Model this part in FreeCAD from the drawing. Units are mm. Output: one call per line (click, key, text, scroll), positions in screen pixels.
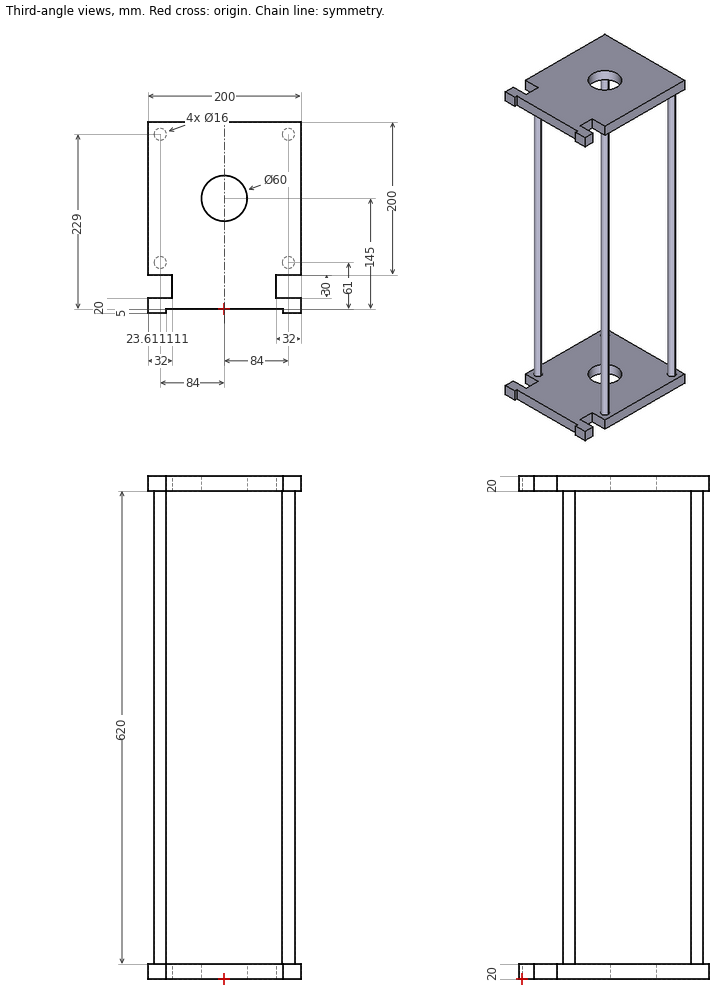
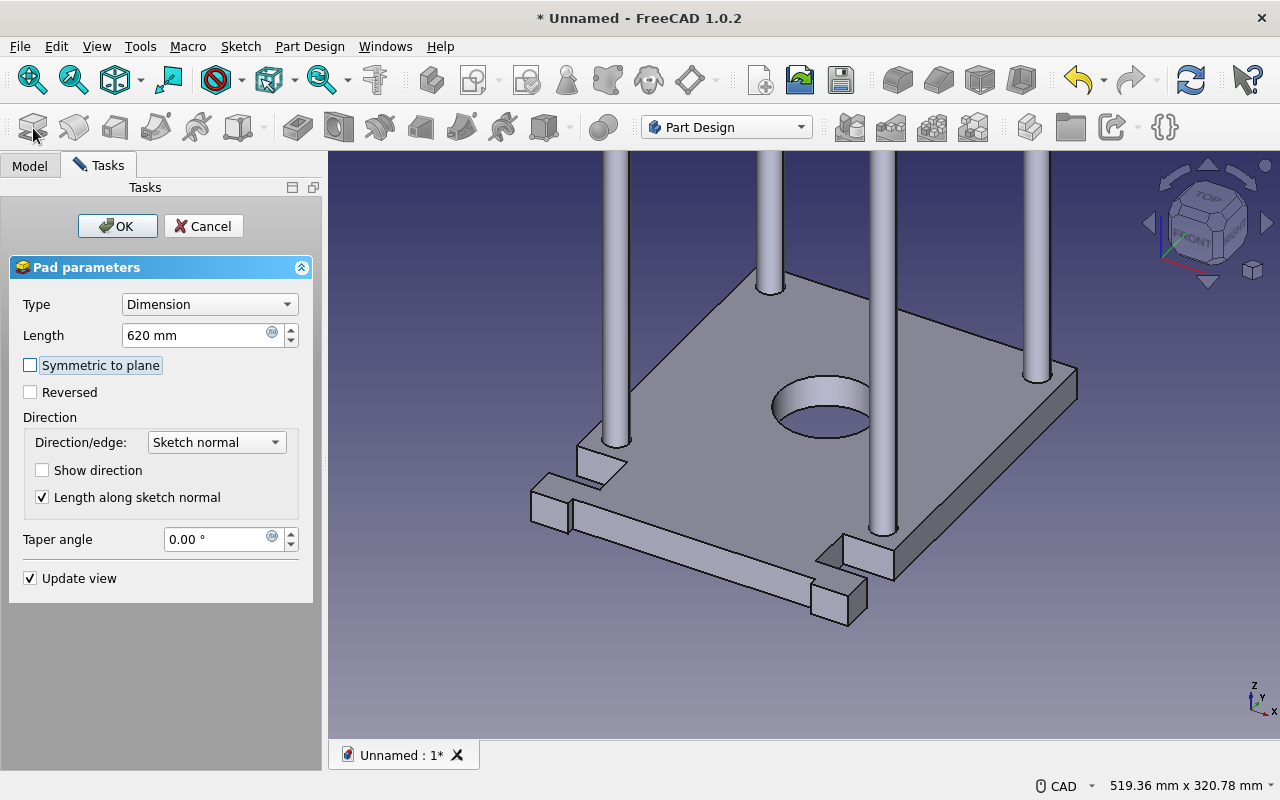
click(118, 226)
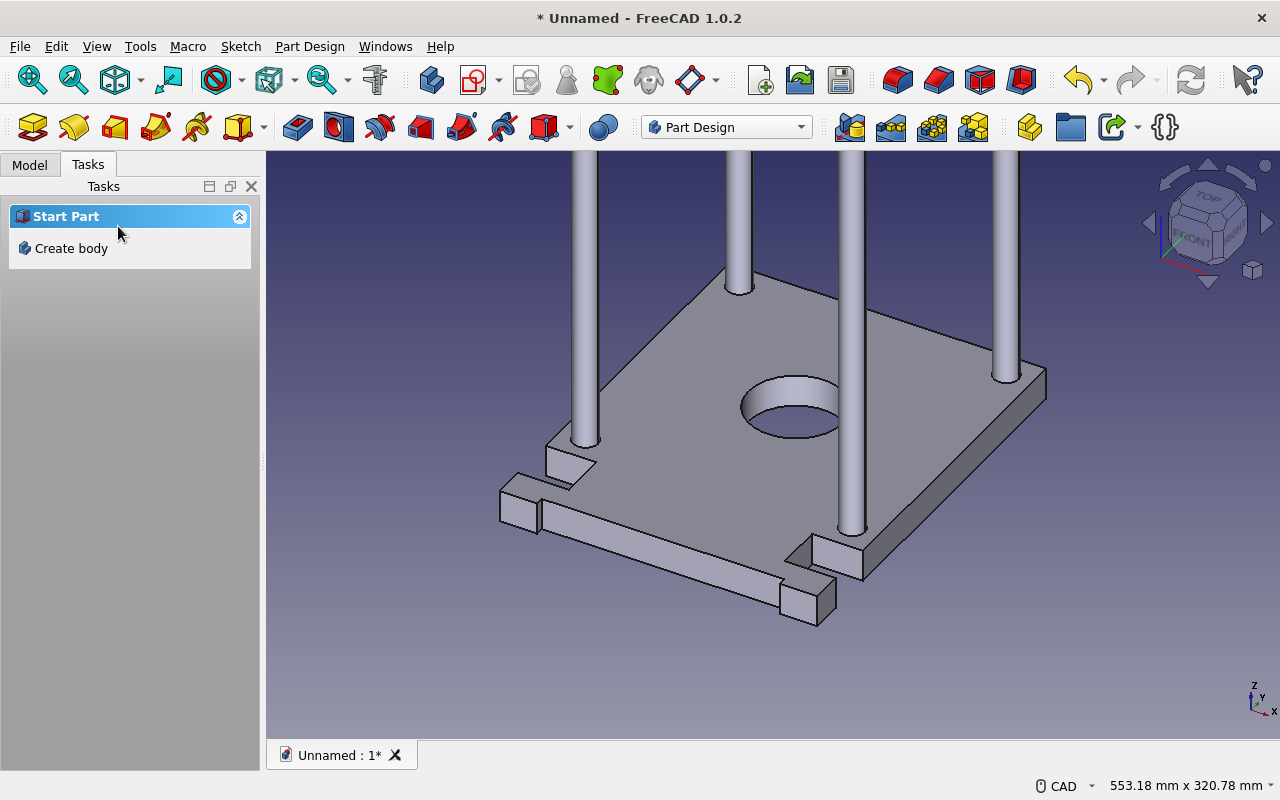
click(33, 80)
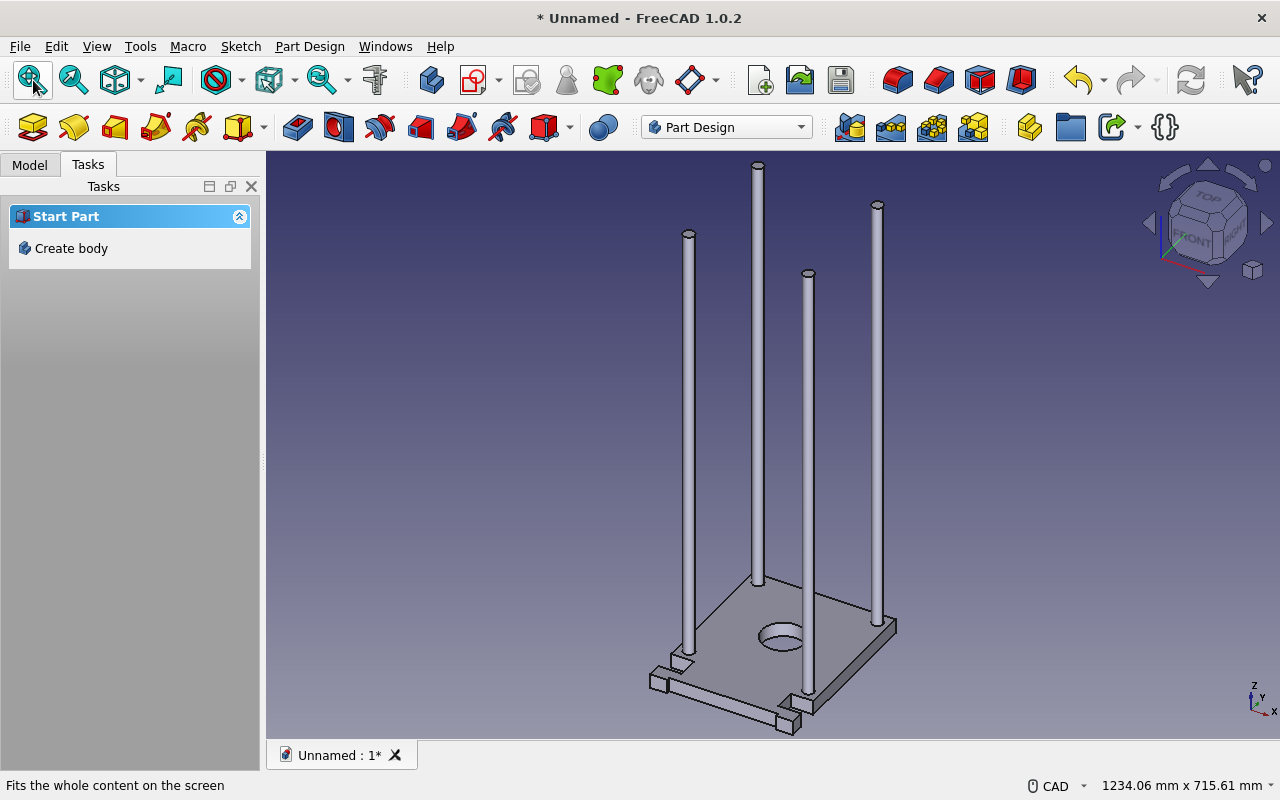
scroll(878, 204, up, 4)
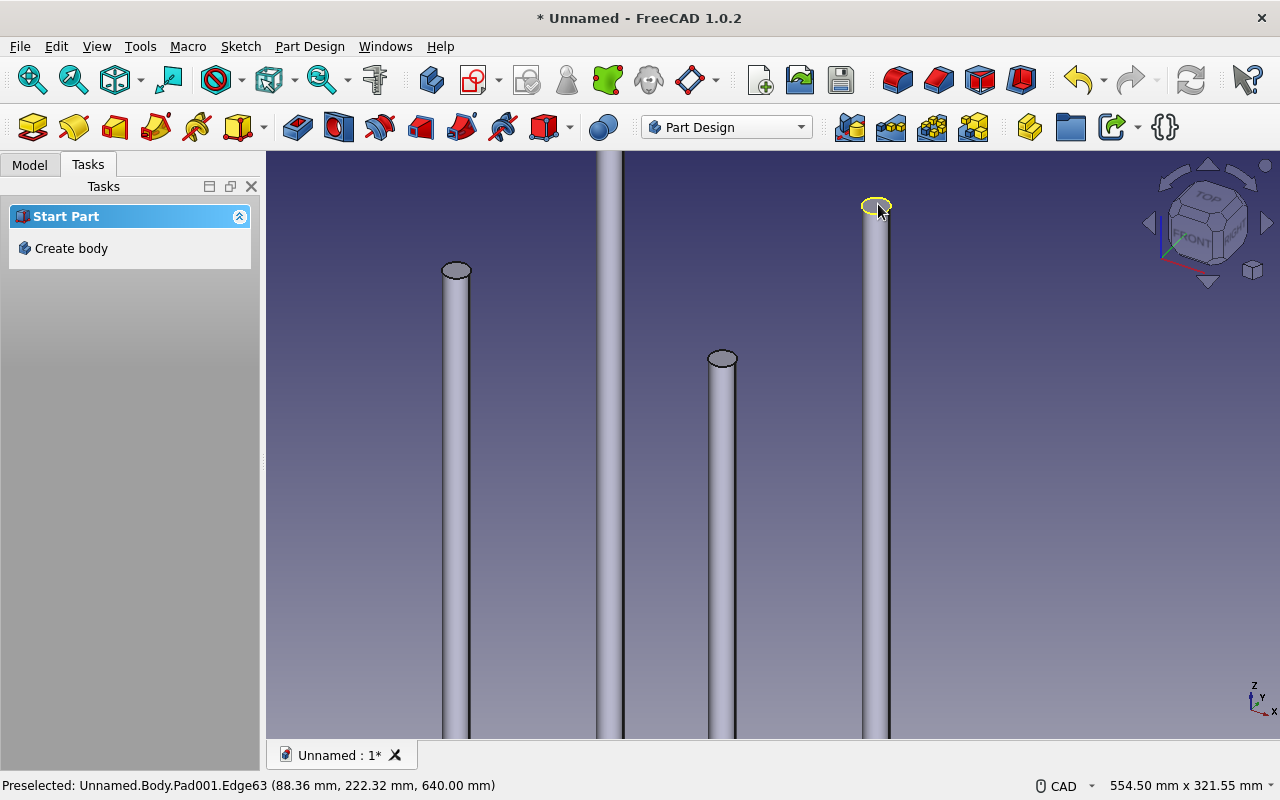
click(876, 205)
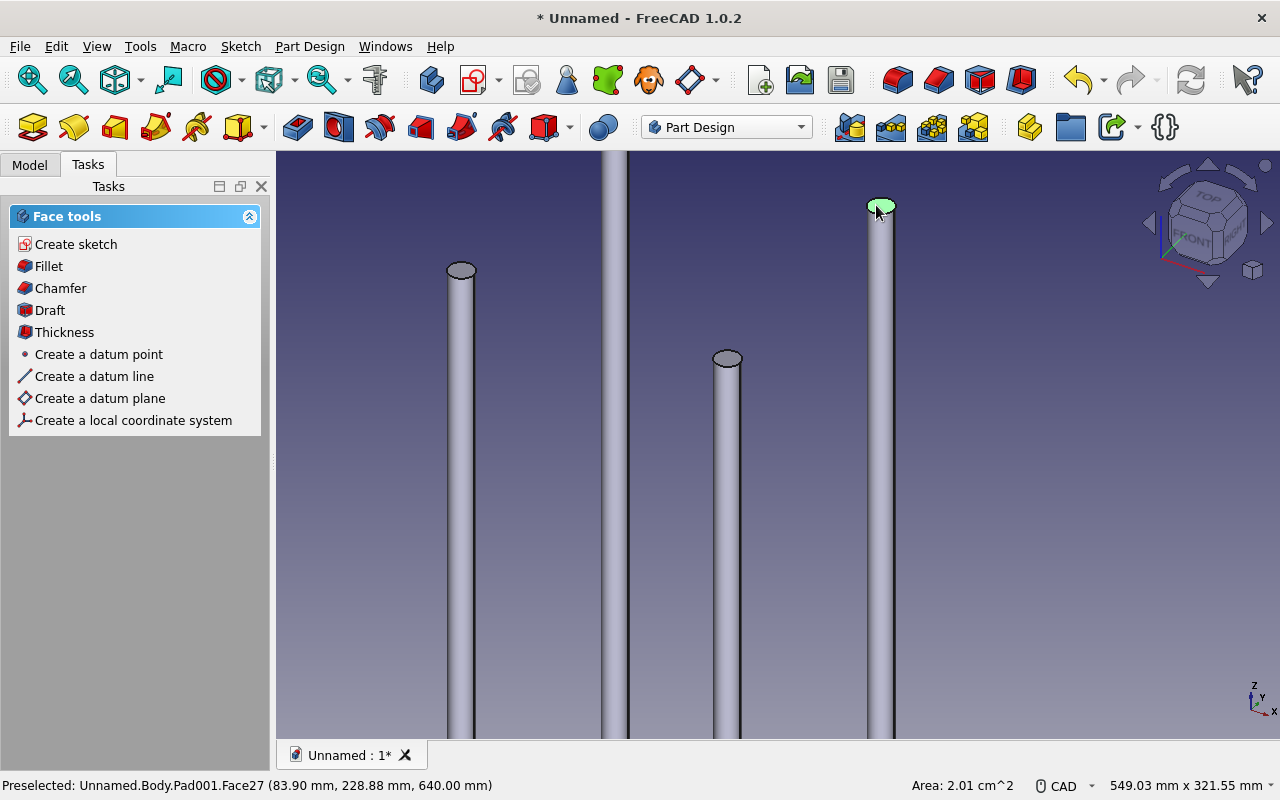
click(472, 80)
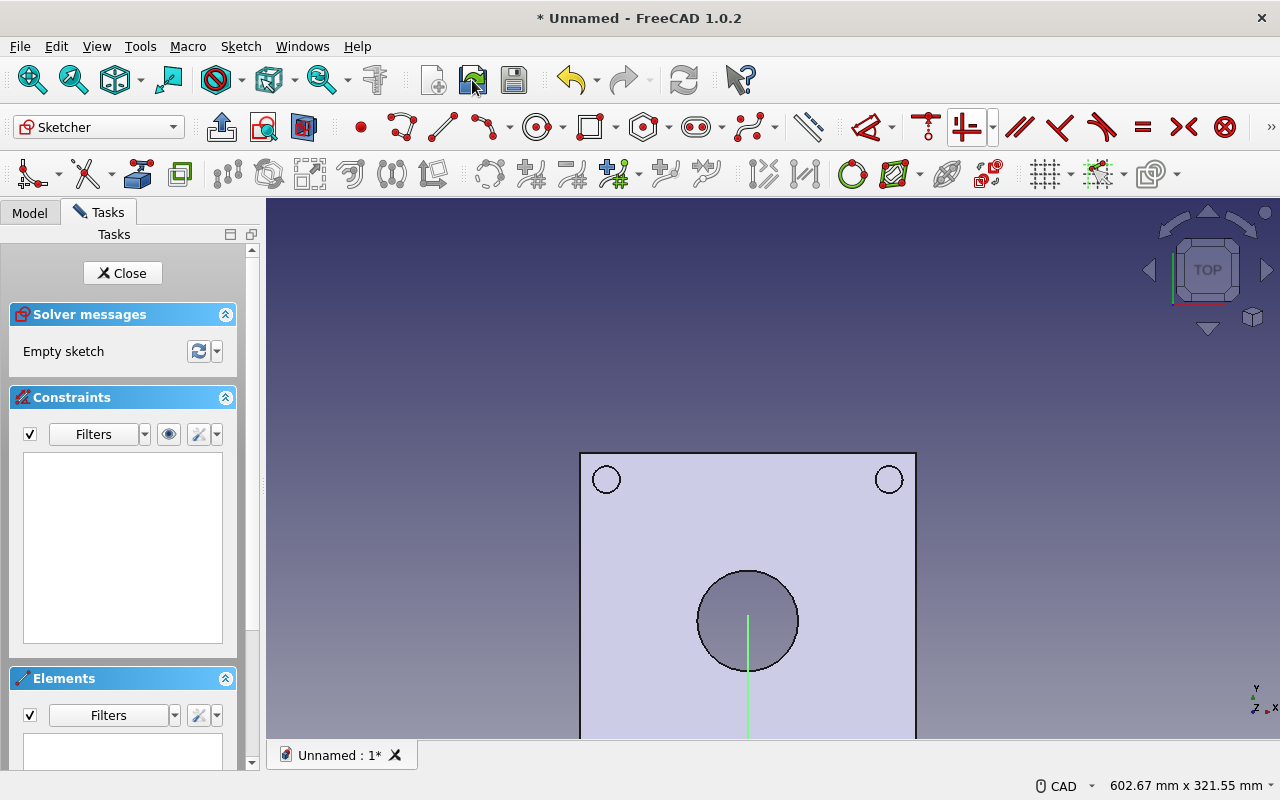
scroll(617, 226, down, 2)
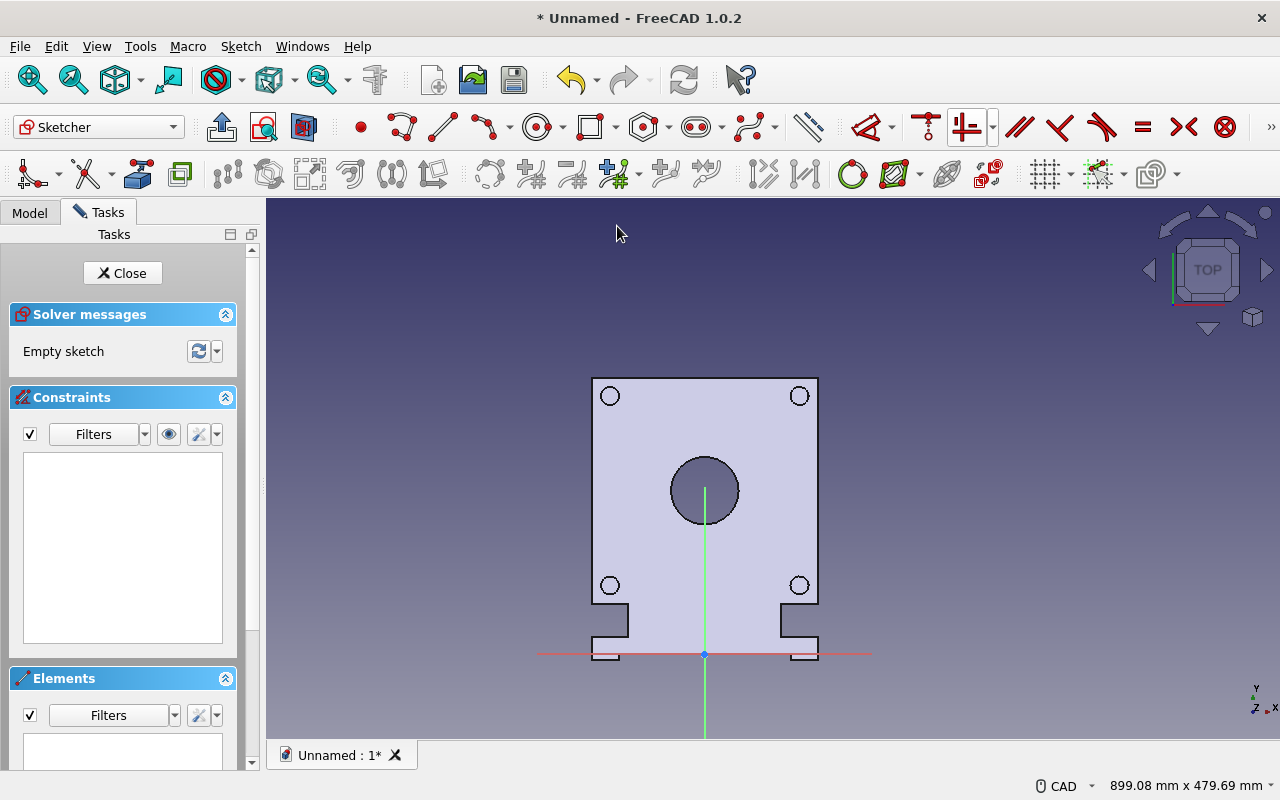
click(402, 128)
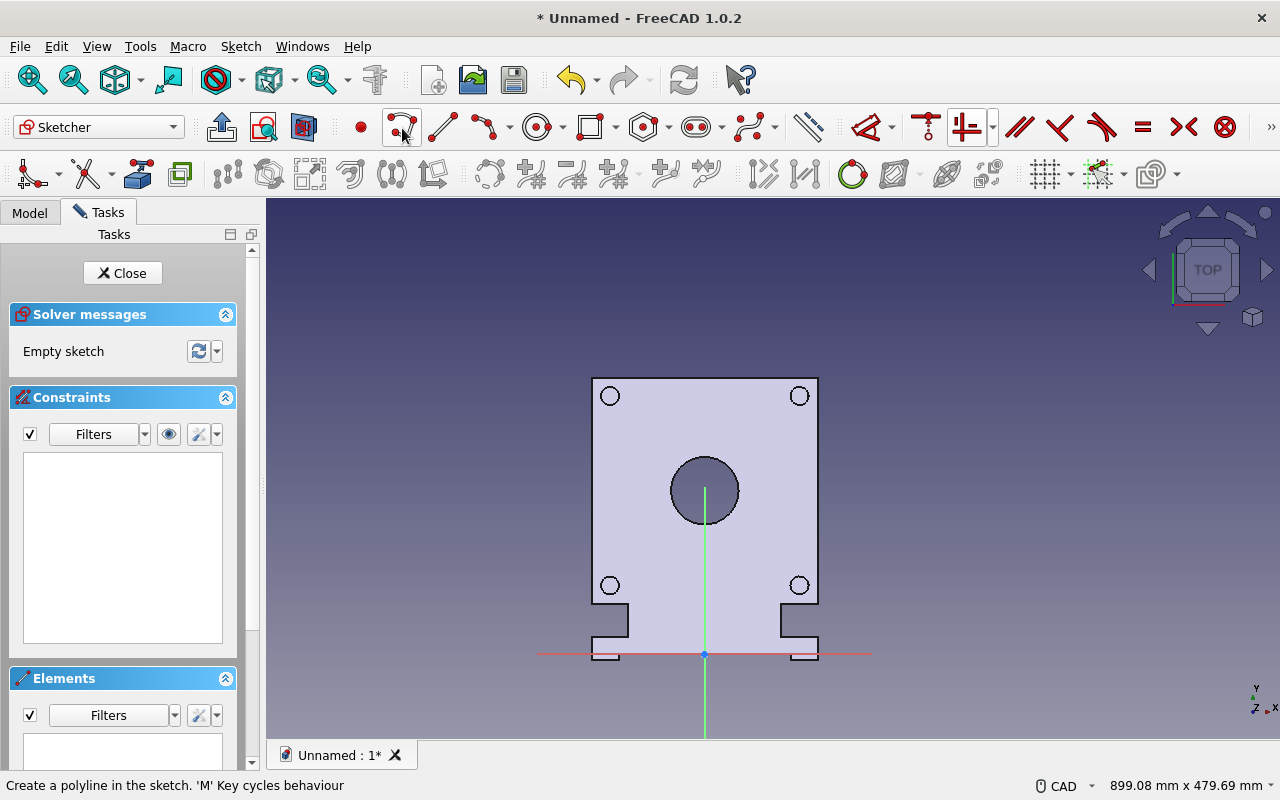
click(781, 637)
click(781, 604)
click(818, 604)
click(818, 378)
click(592, 378)
click(592, 604)
click(628, 604)
click(628, 637)
click(592, 637)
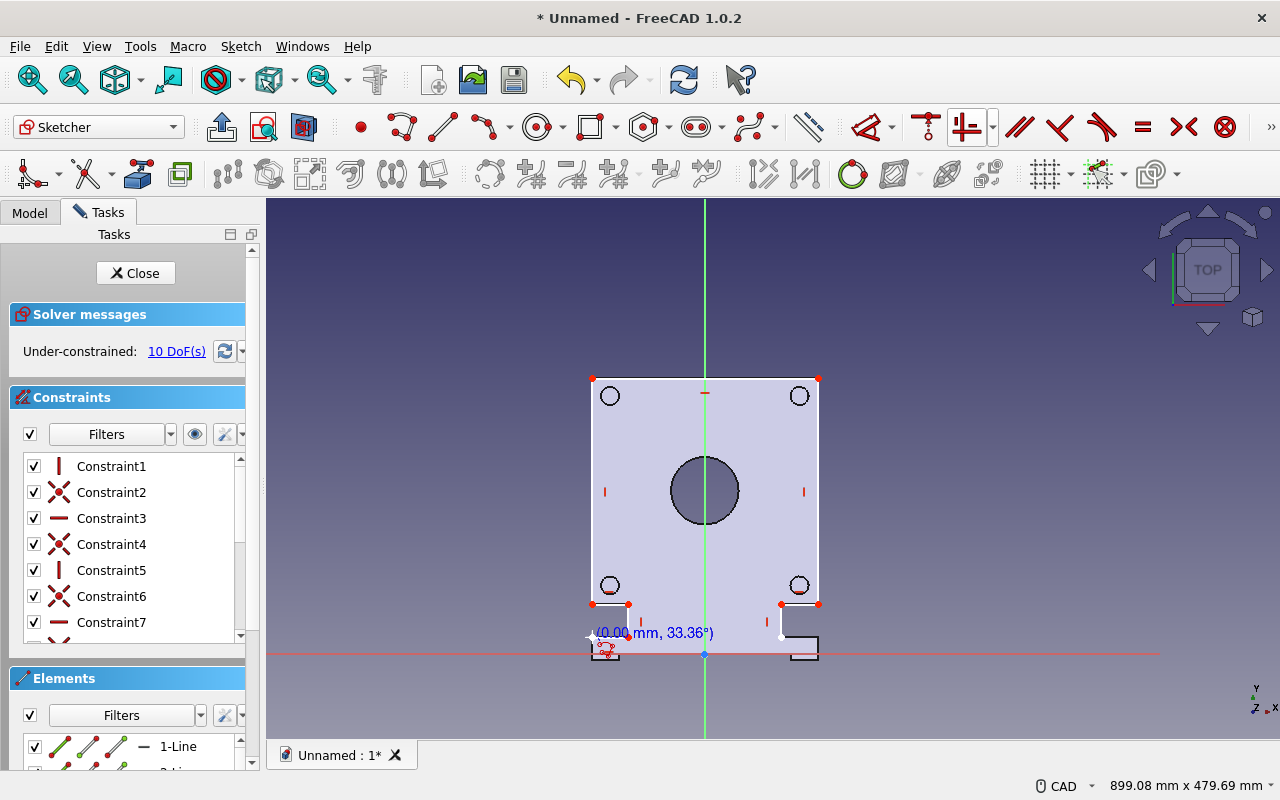
scroll(592, 660, up, 6)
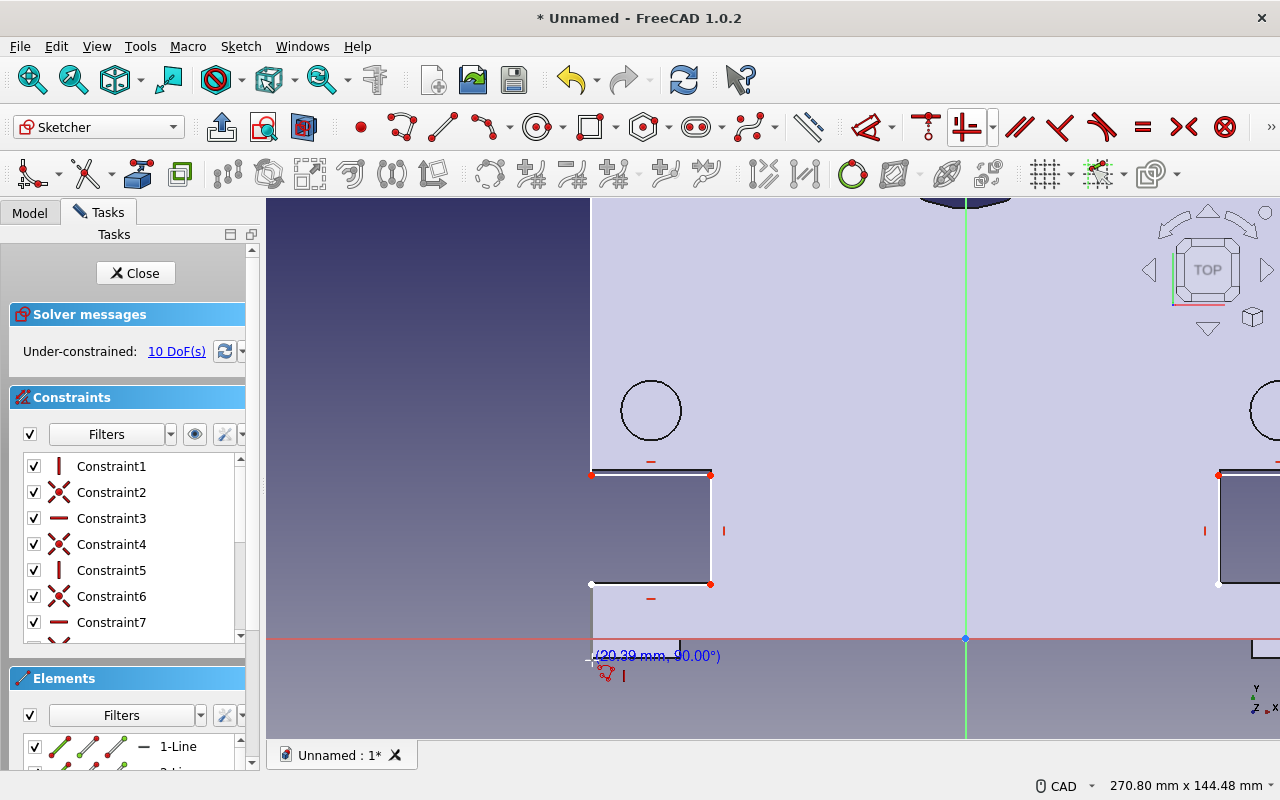
click(591, 658)
click(680, 658)
click(680, 639)